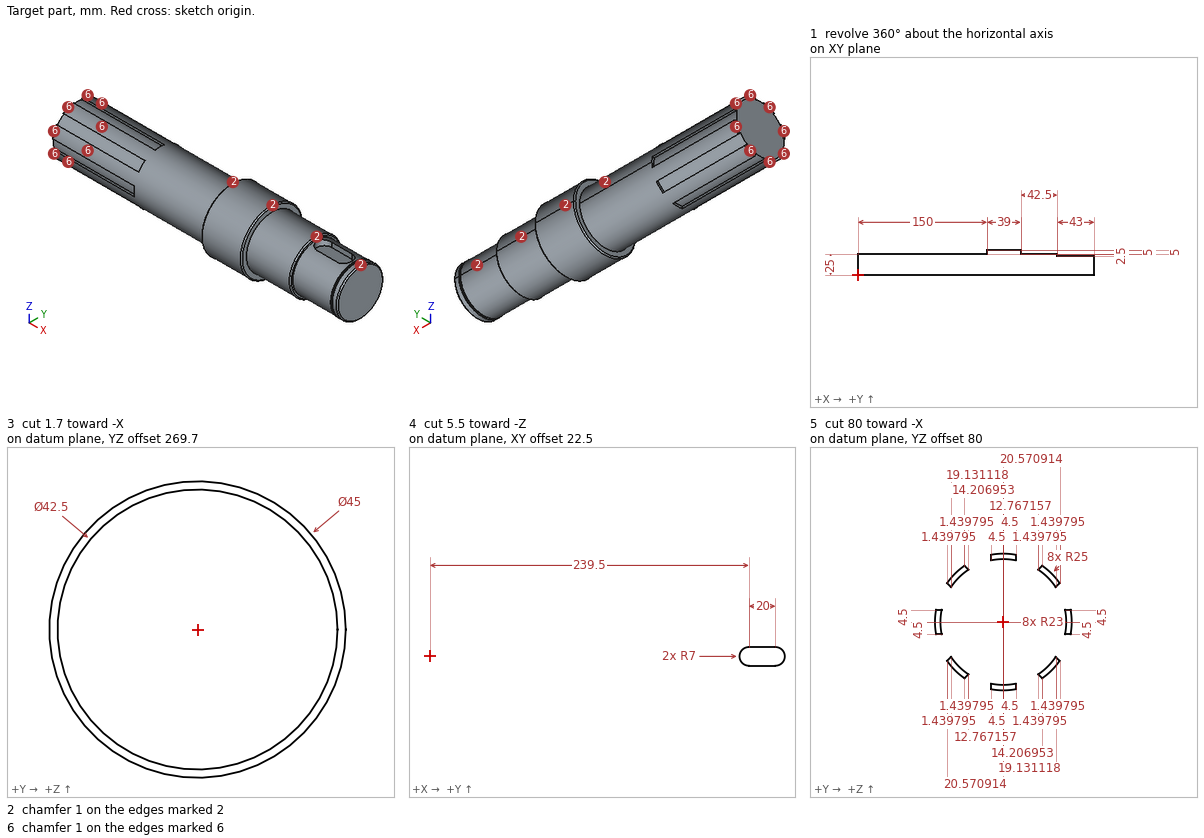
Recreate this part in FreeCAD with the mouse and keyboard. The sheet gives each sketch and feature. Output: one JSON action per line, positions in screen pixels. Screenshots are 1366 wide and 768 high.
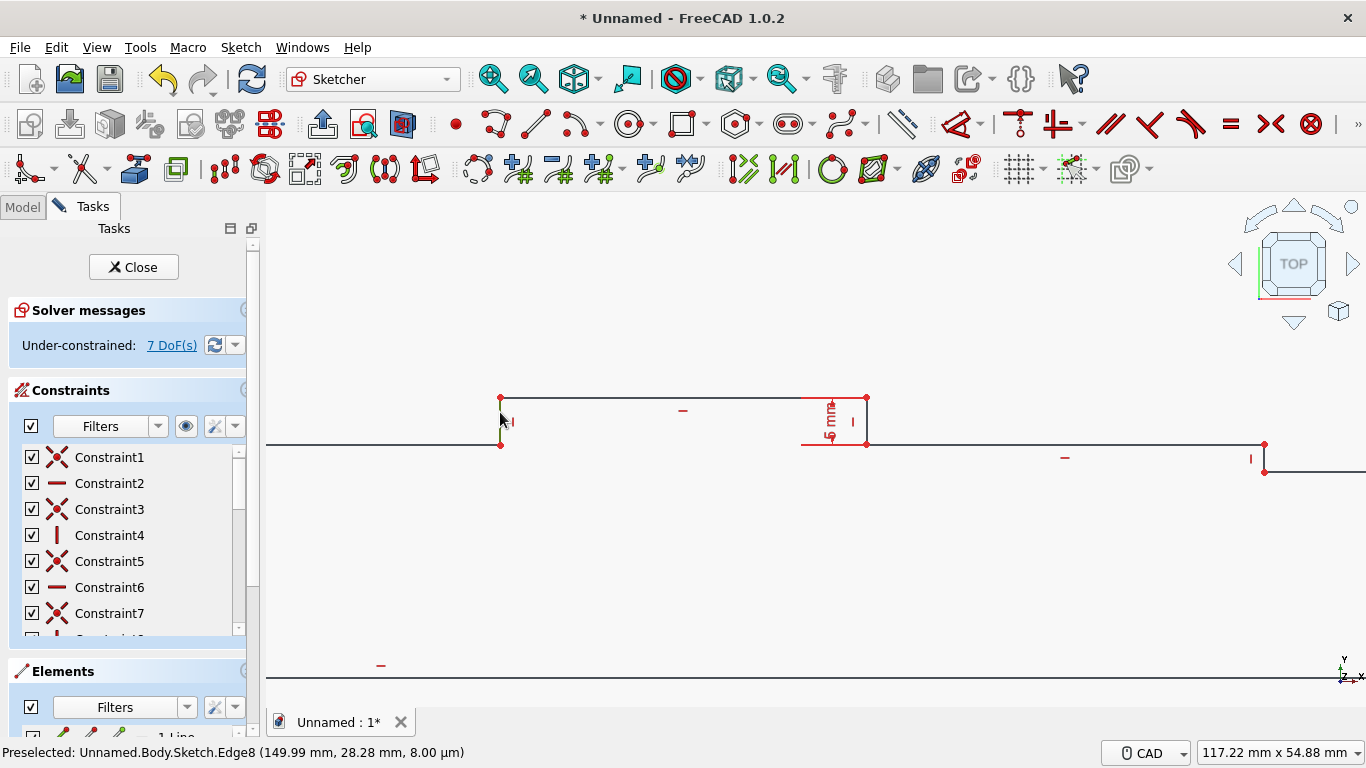
{"action": "key", "text": "i"}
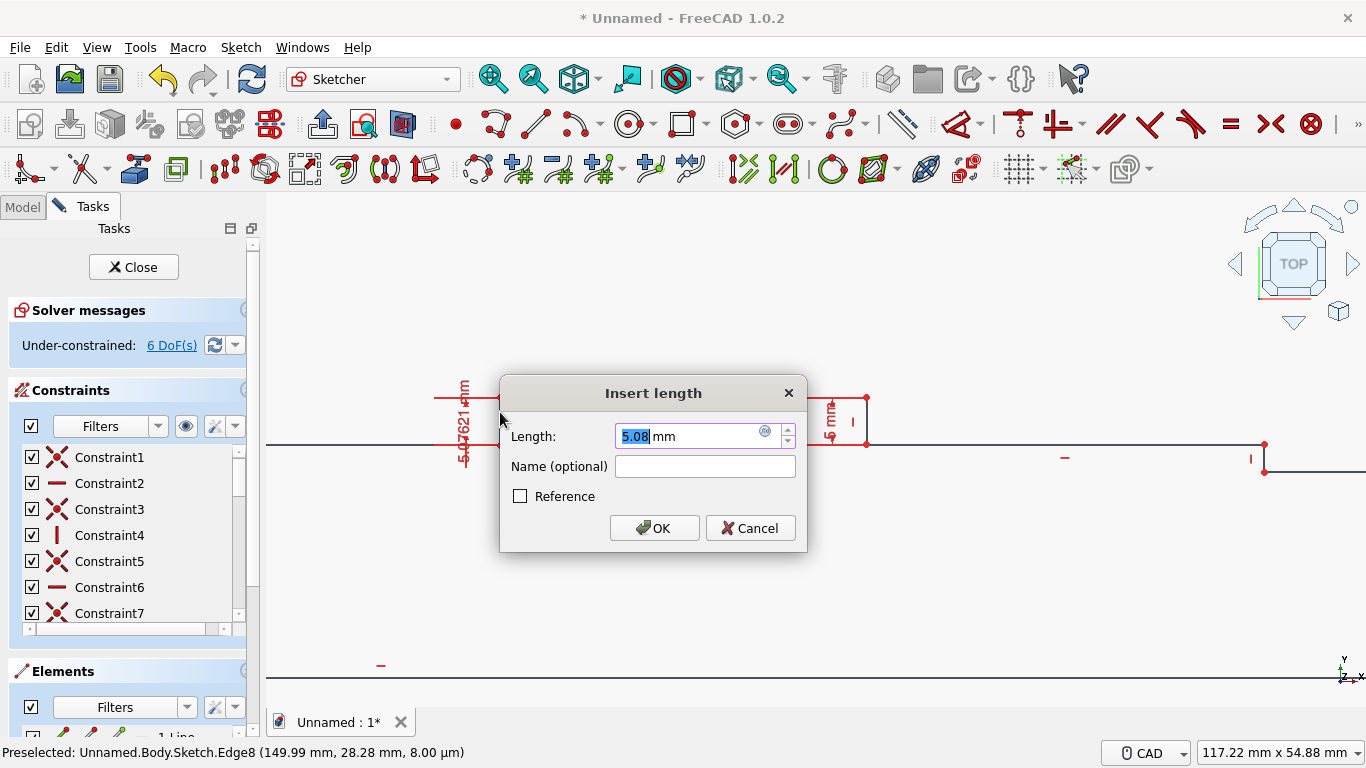
{"action": "type", "text": "5"}
{"action": "key", "text": "Return"}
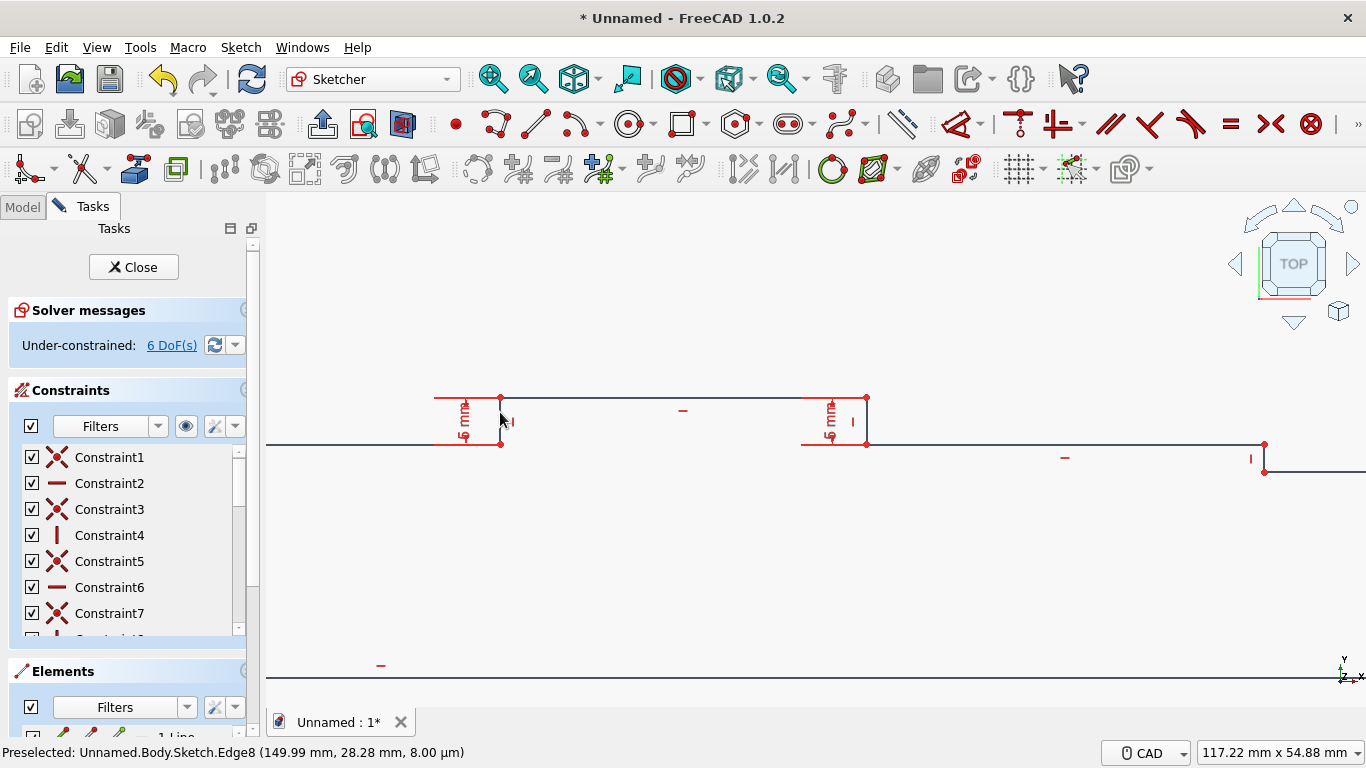
{"action": "scroll", "coordinate": [868, 421], "scroll_direction": "down", "scroll_amount": 7}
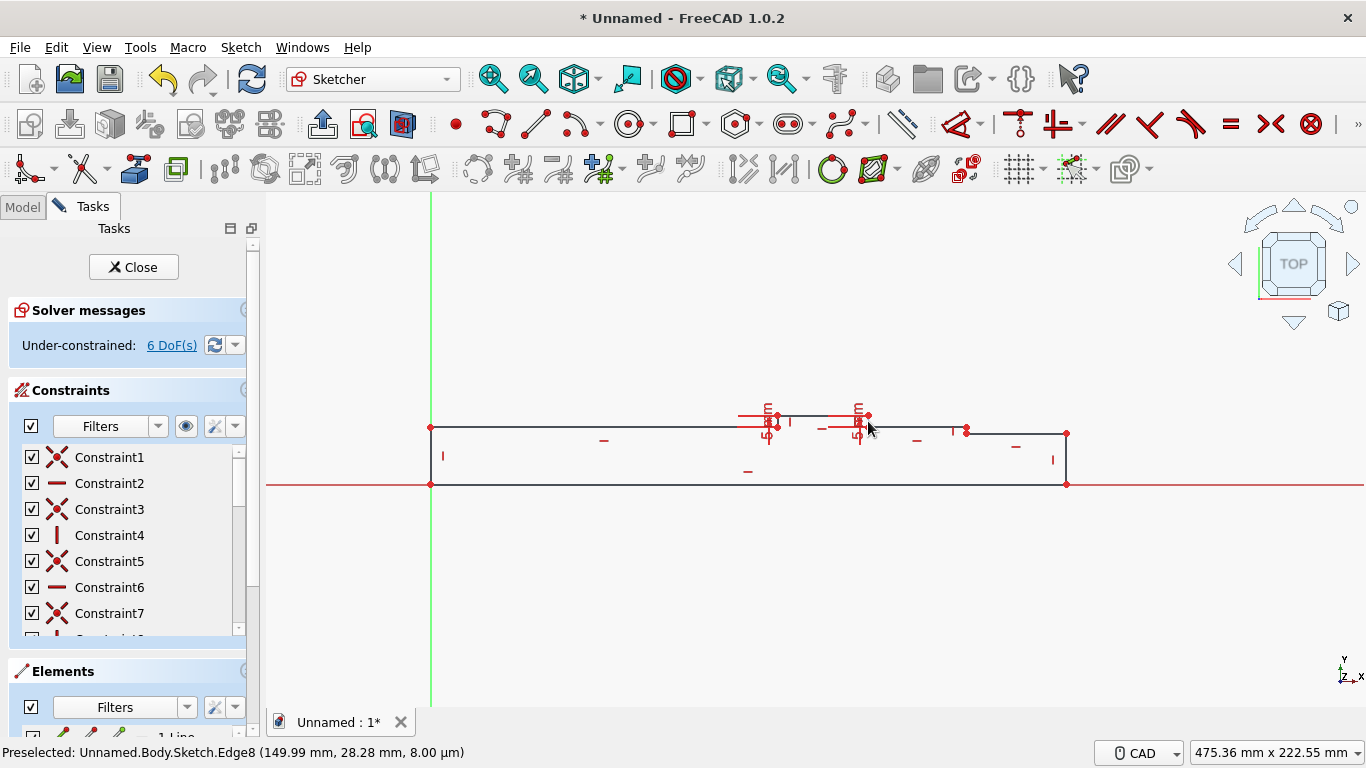
{"action": "left_click", "coordinate": [1036, 434]}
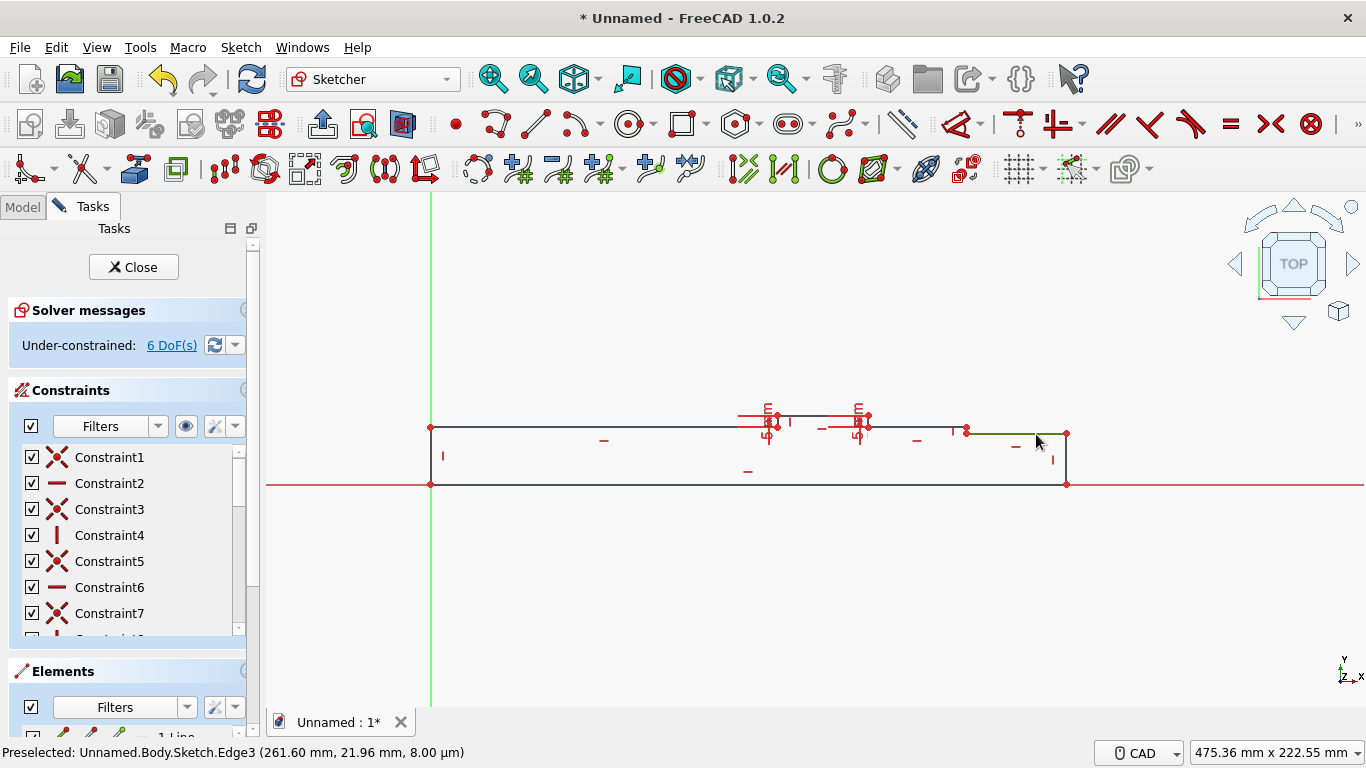
{"action": "key", "text": "l"}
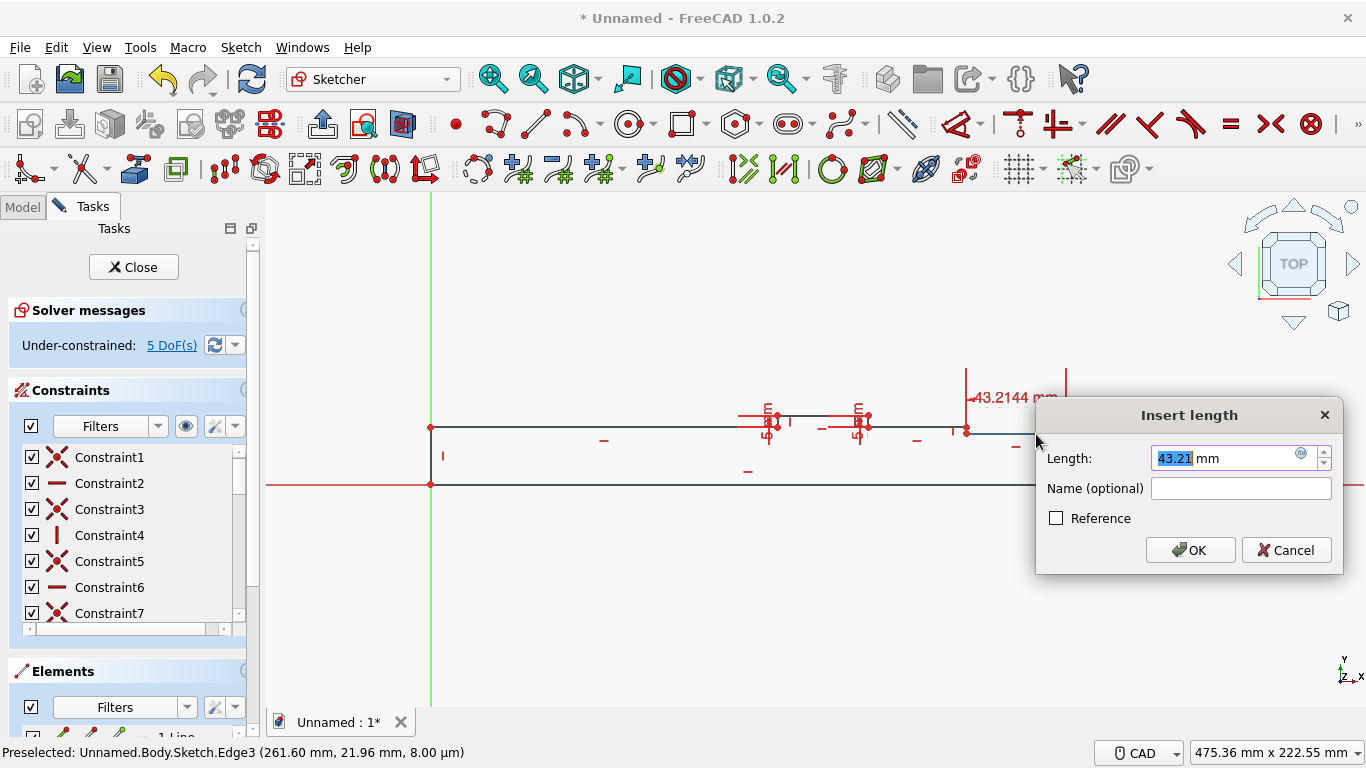
{"action": "type", "text": "43"}
{"action": "key", "text": "Return"}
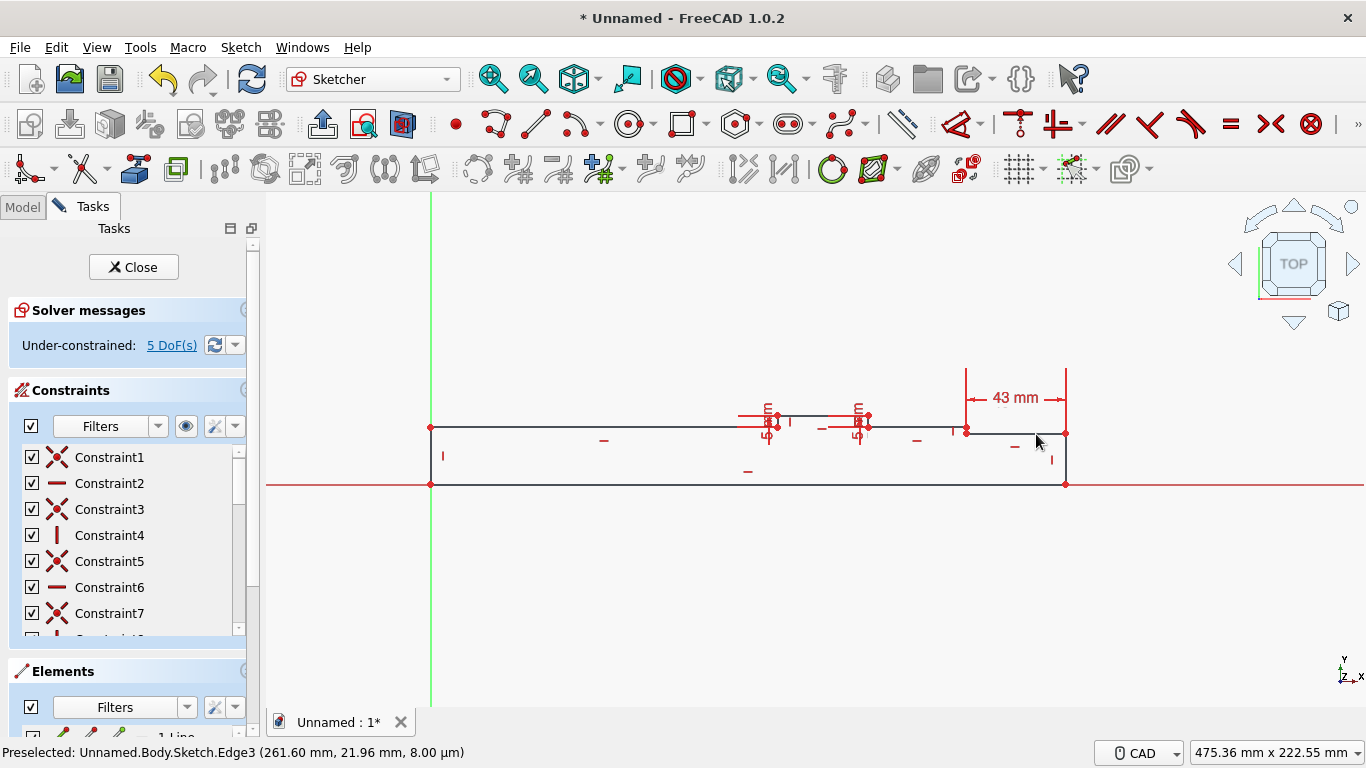
{"action": "left_click", "coordinate": [841, 416]}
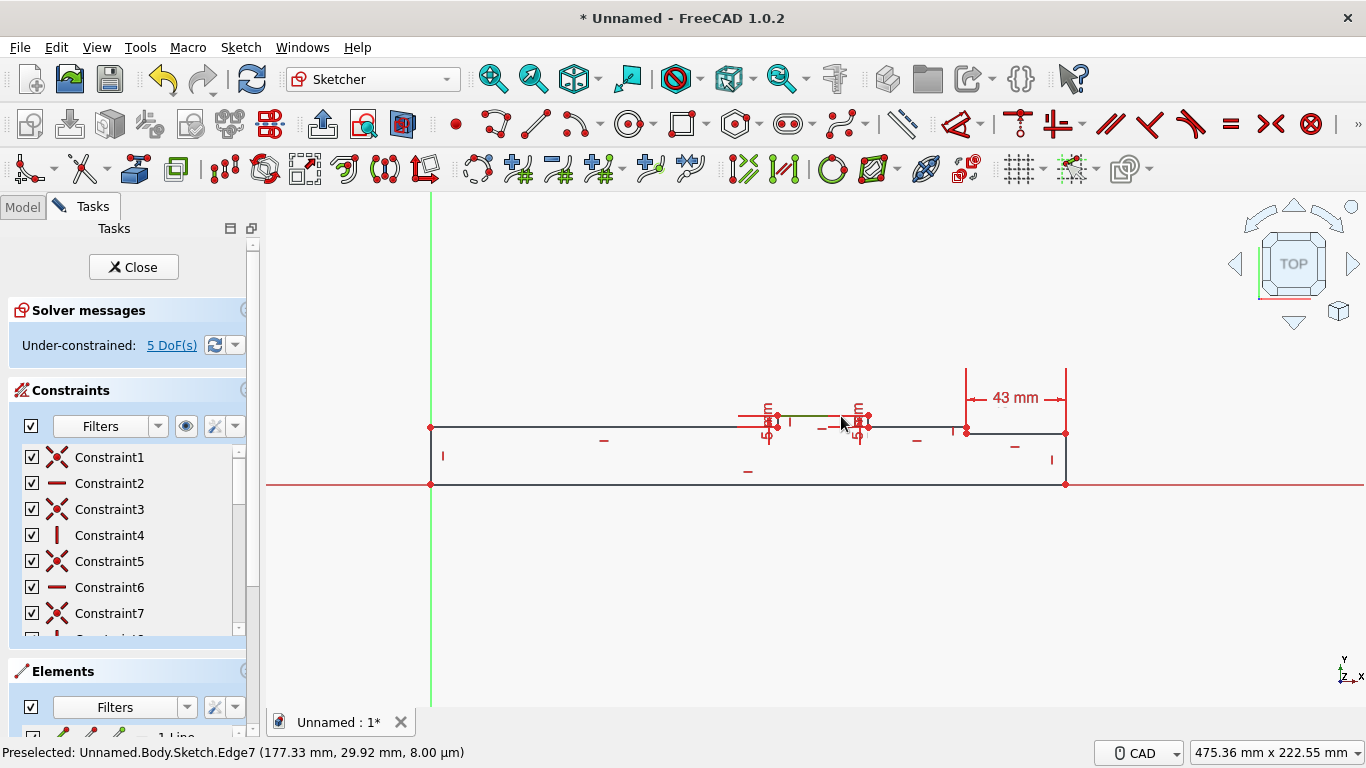
{"action": "key", "text": "l"}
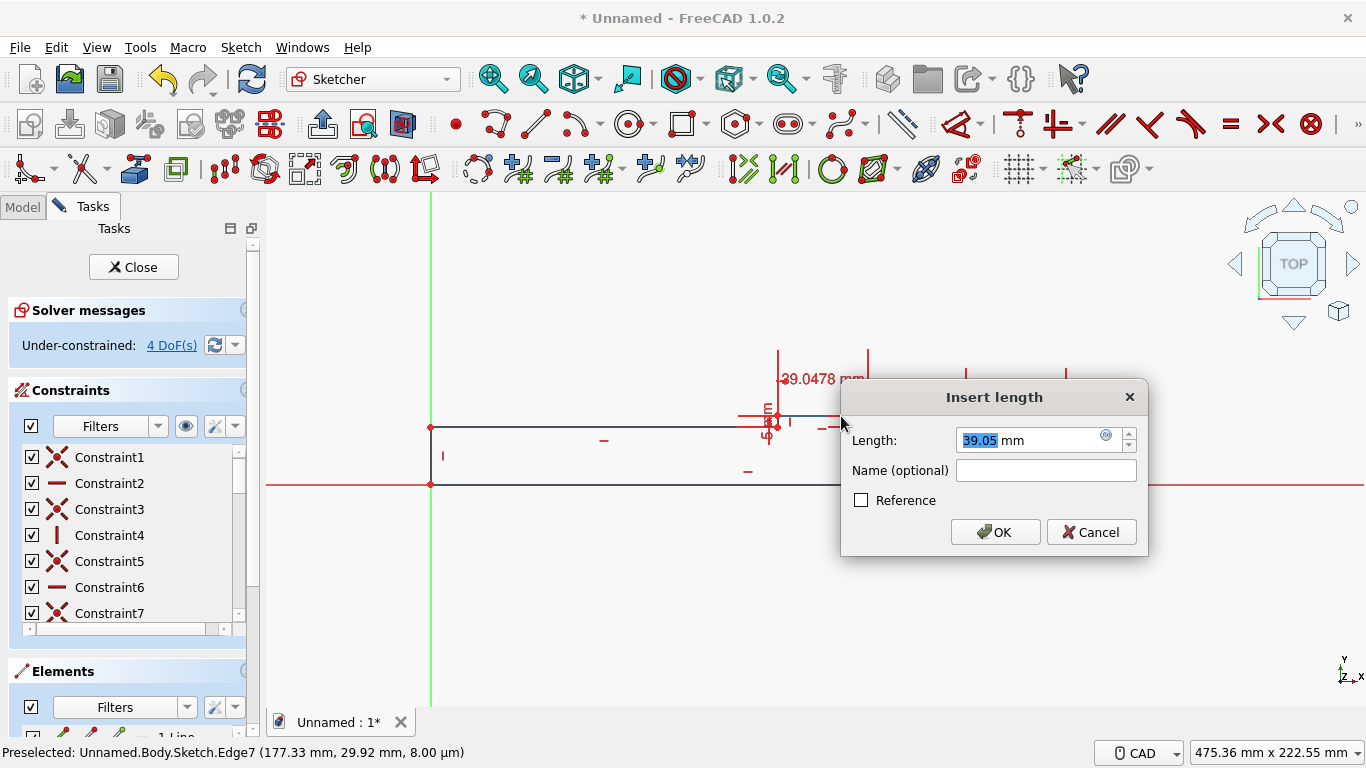
{"action": "type", "text": "39"}
{"action": "key", "text": "Return"}